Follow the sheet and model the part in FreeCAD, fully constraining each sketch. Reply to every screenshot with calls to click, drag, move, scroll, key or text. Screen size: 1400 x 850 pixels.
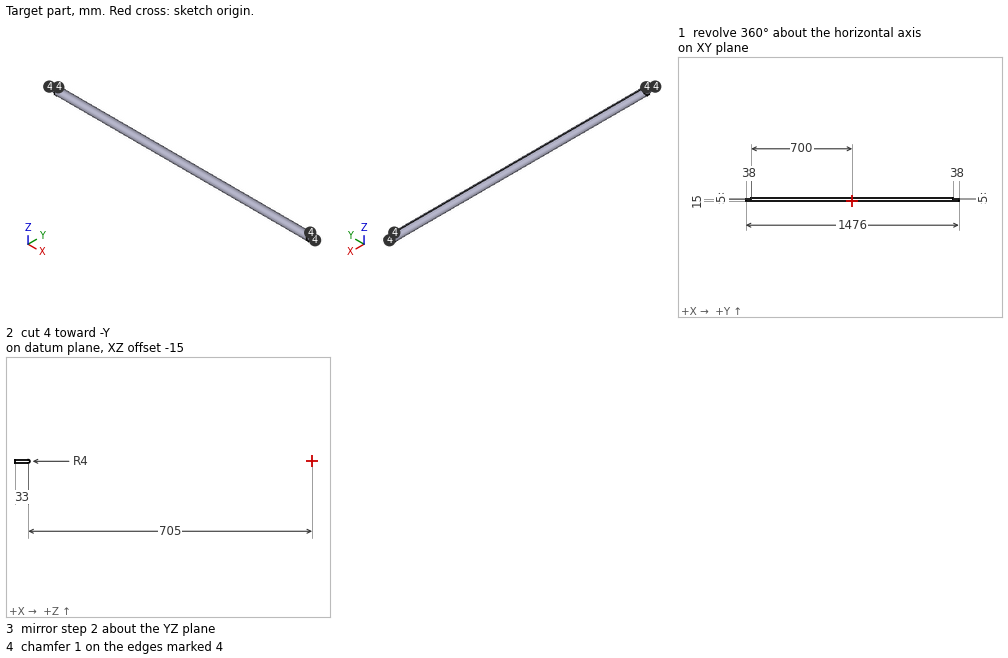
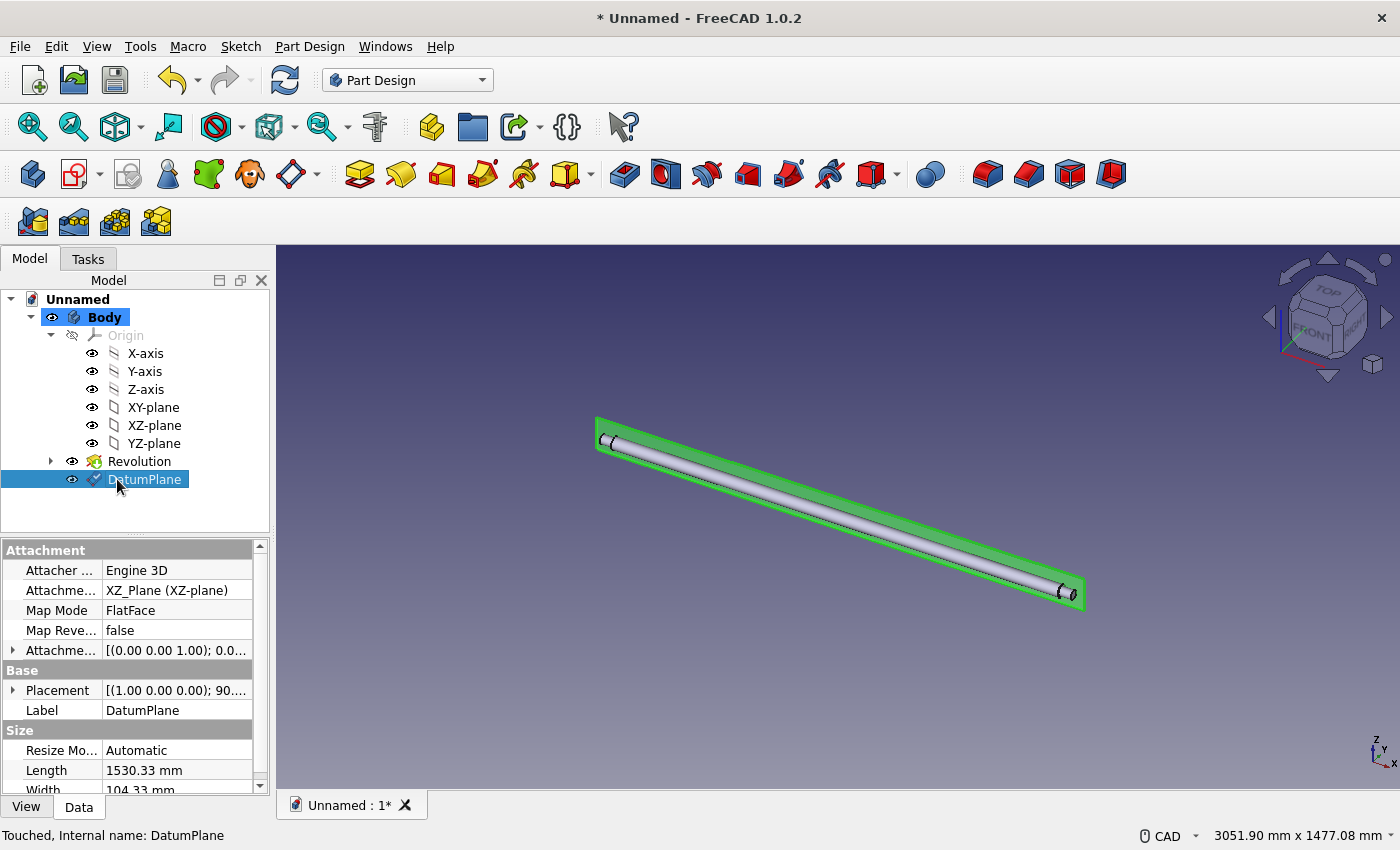
click(74, 174)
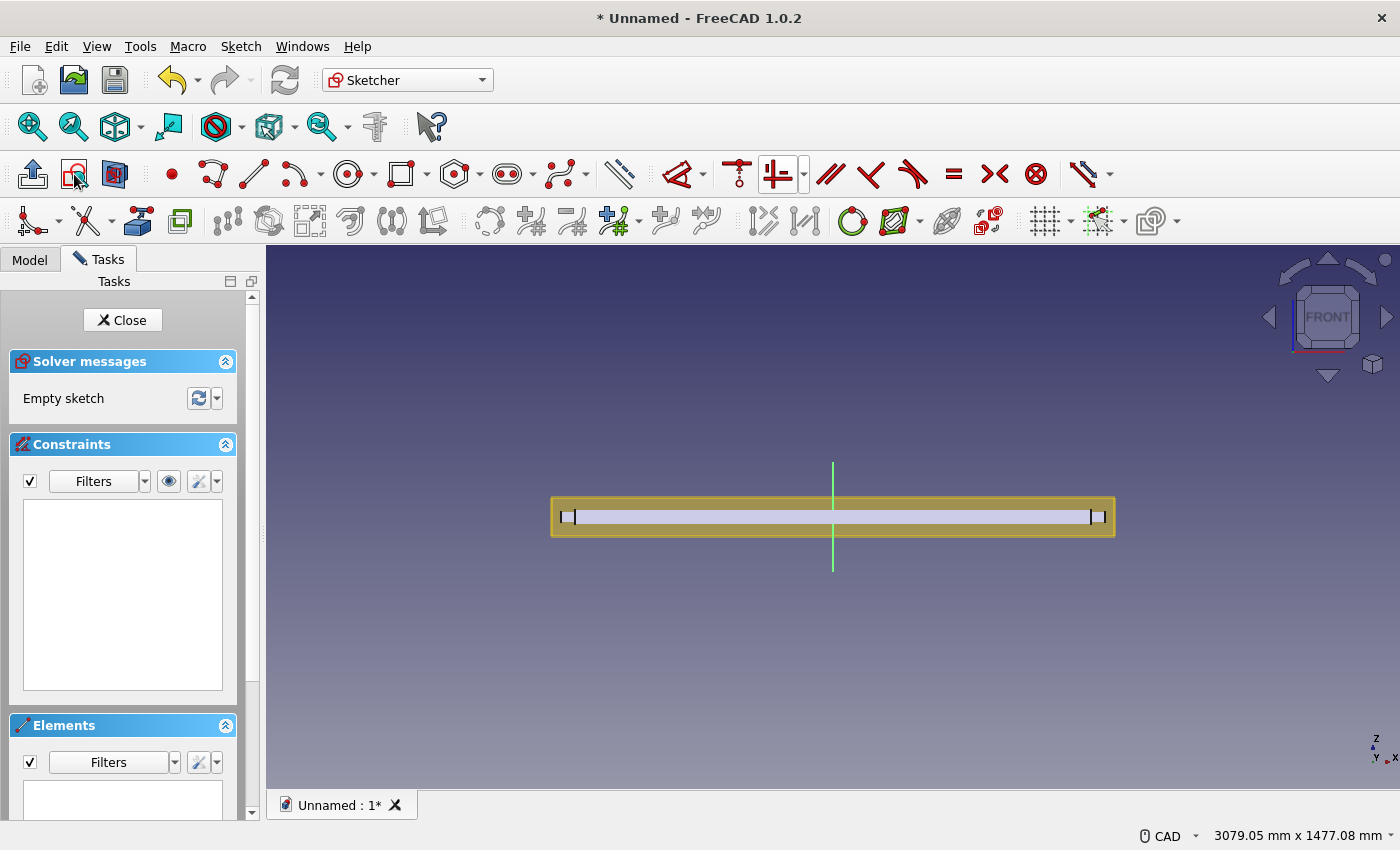
click(115, 174)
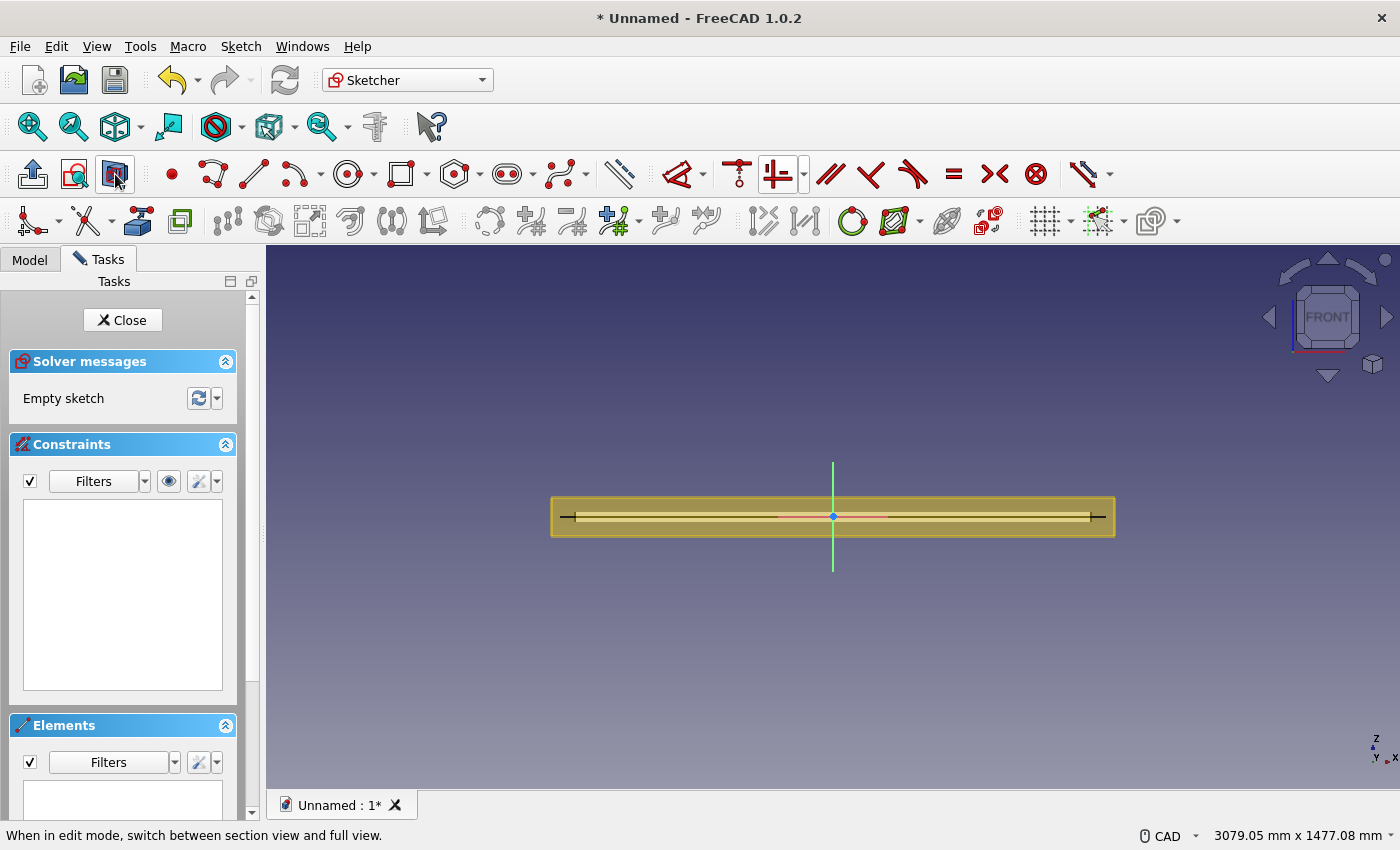
scroll(558, 517, up, 15)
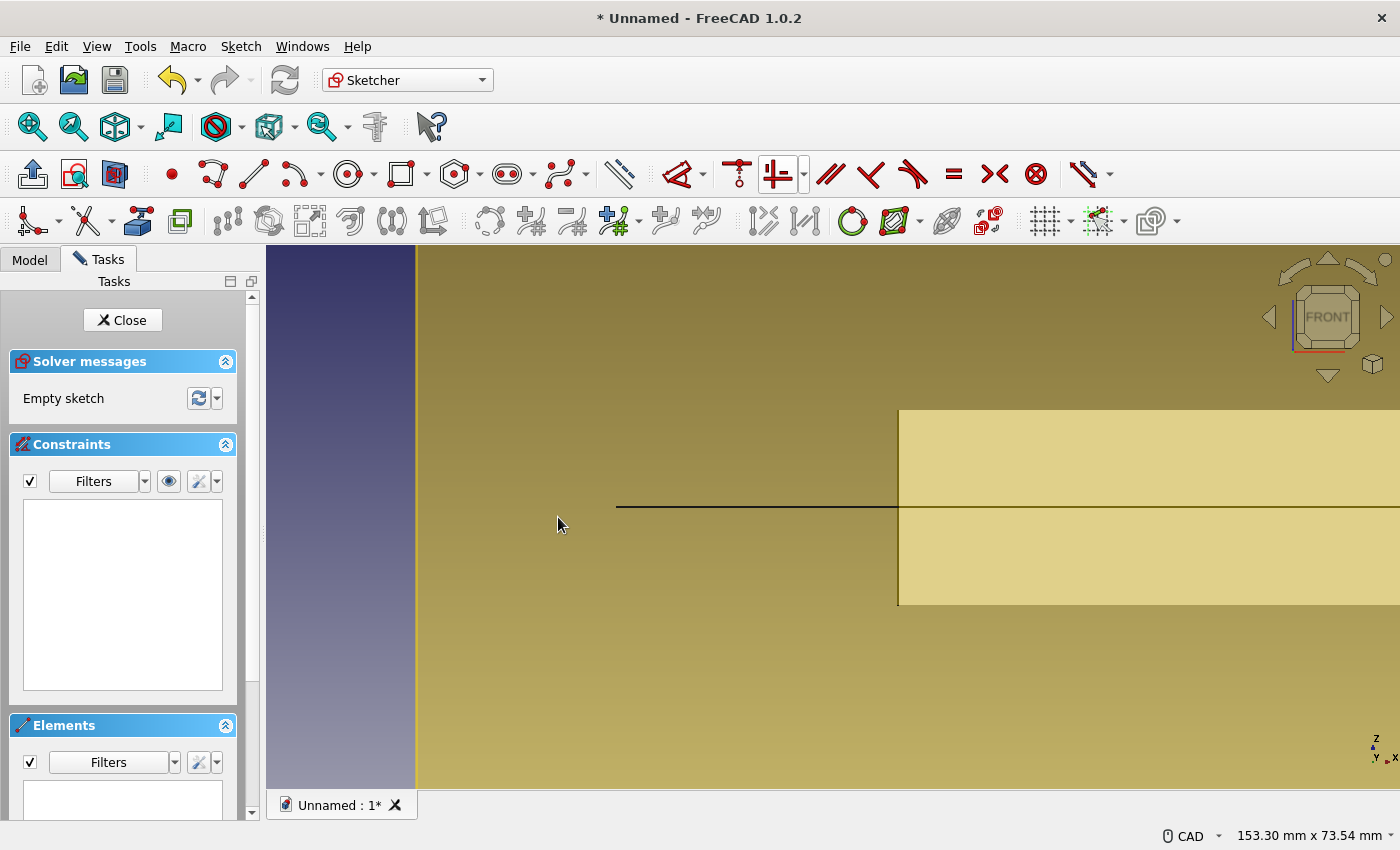
scroll(746, 500, up, 4)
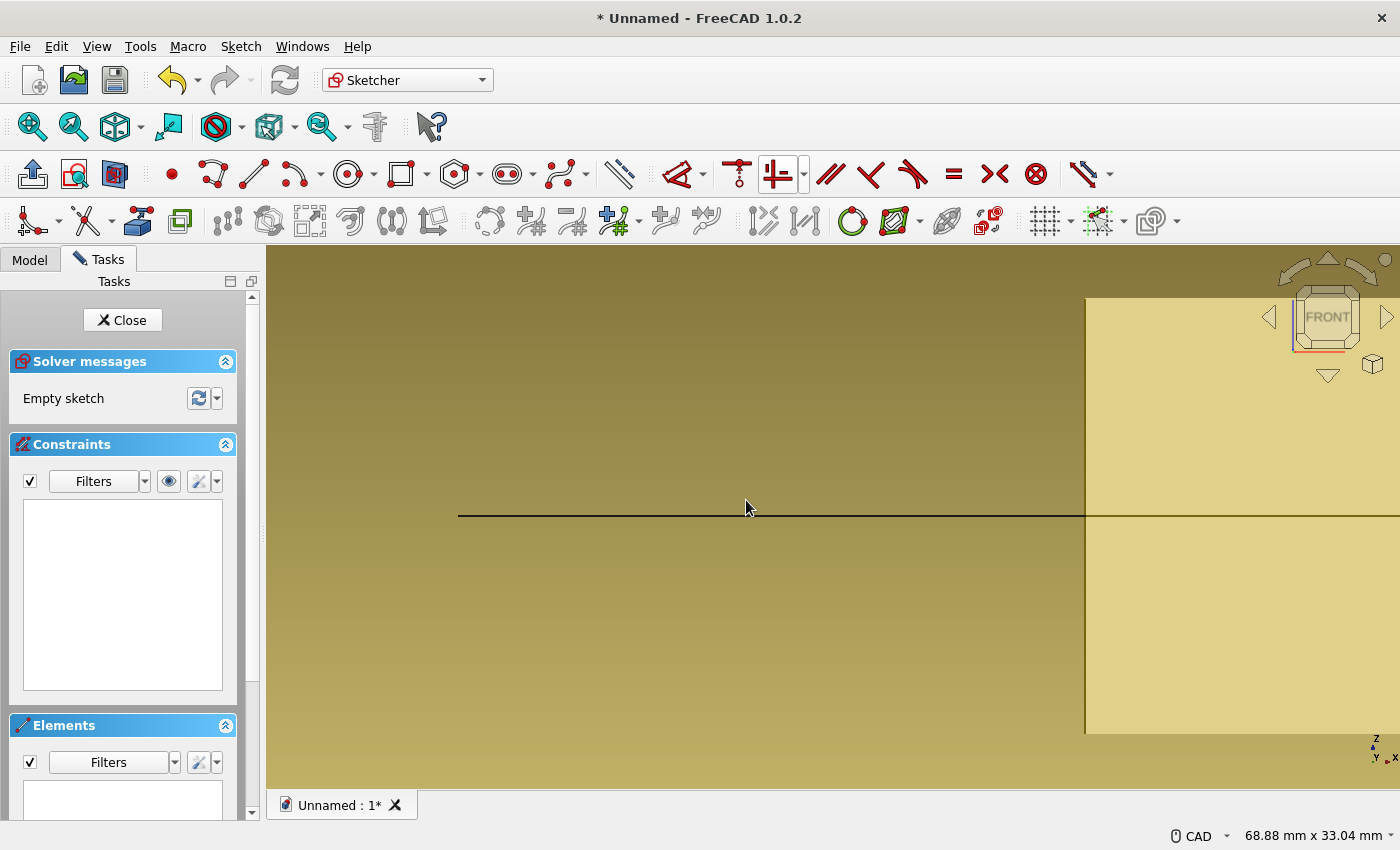
click(213, 174)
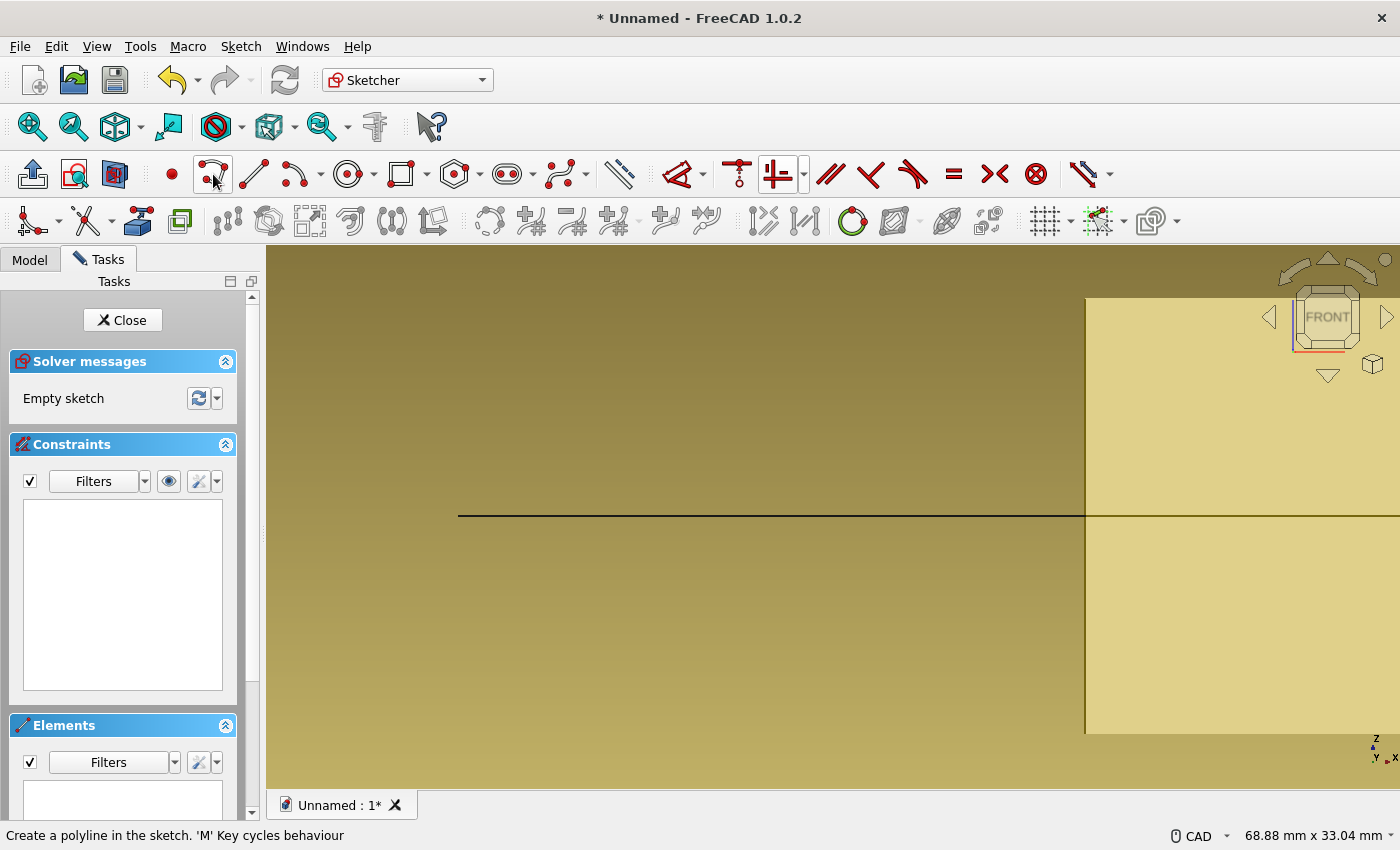
click(1002, 582)
click(459, 582)
click(459, 450)
click(1002, 450)
right_click(1002, 450)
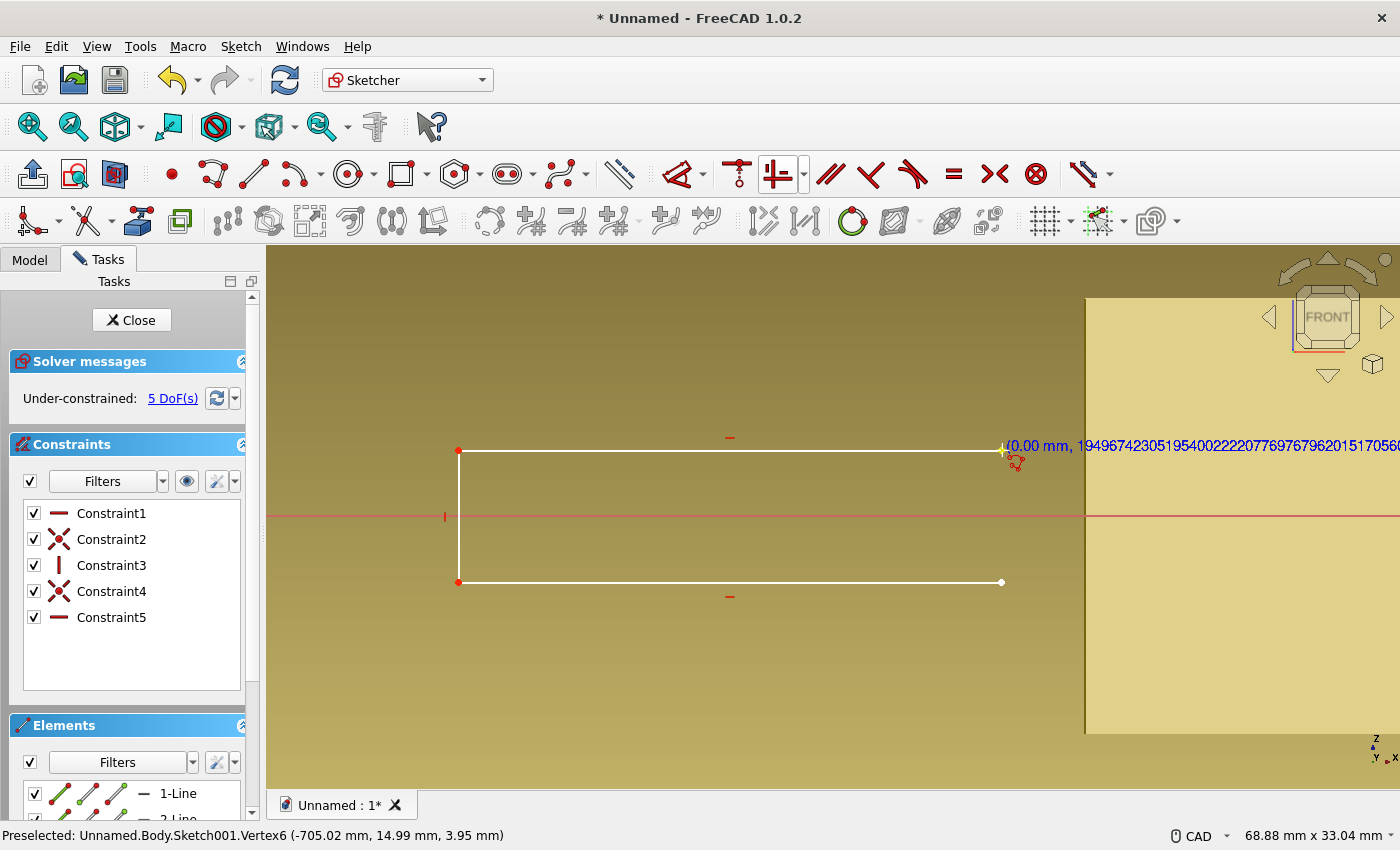
key(g)
key(3)
key(a)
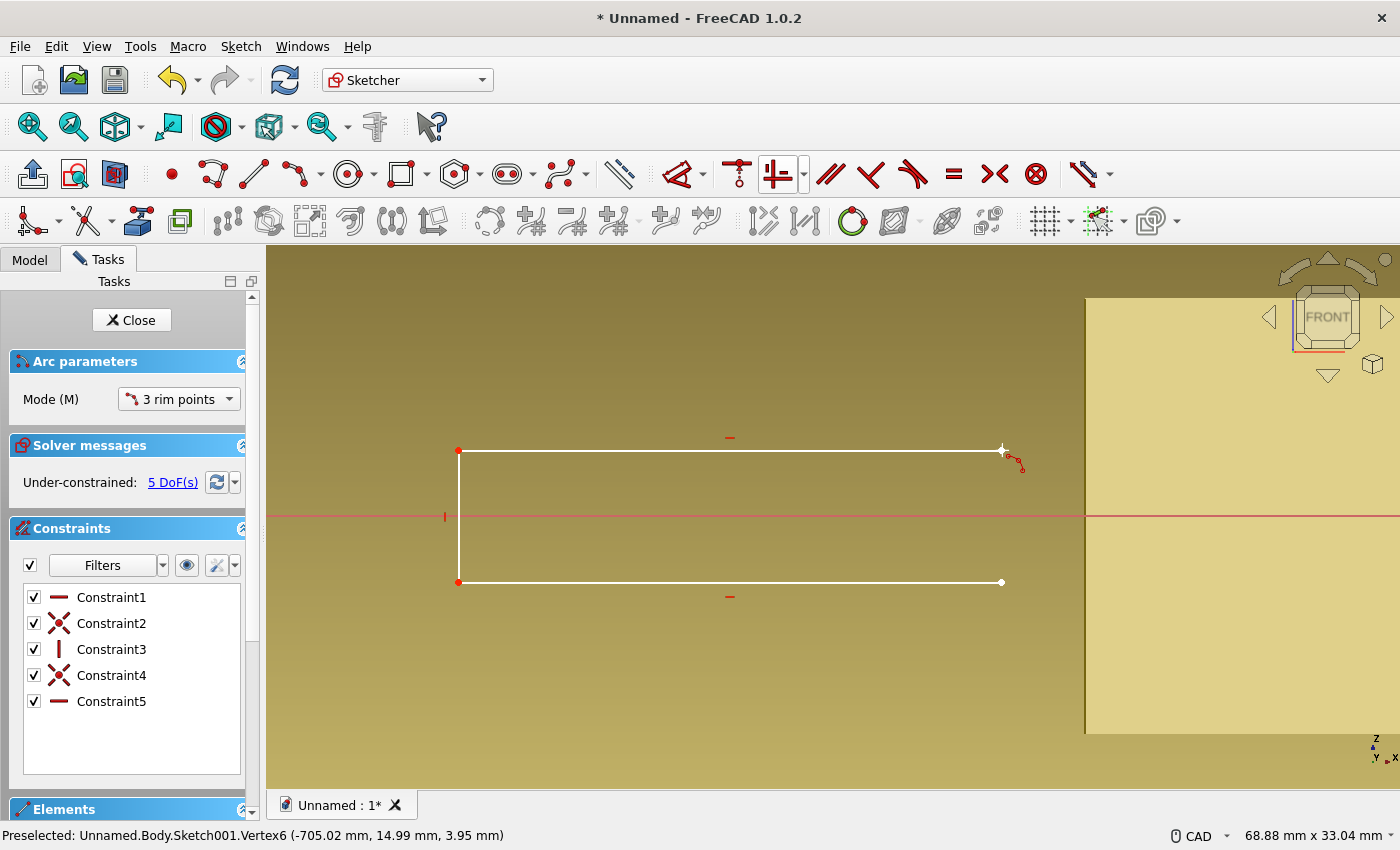
click(1002, 451)
click(1002, 583)
click(1065, 536)
key(Escape)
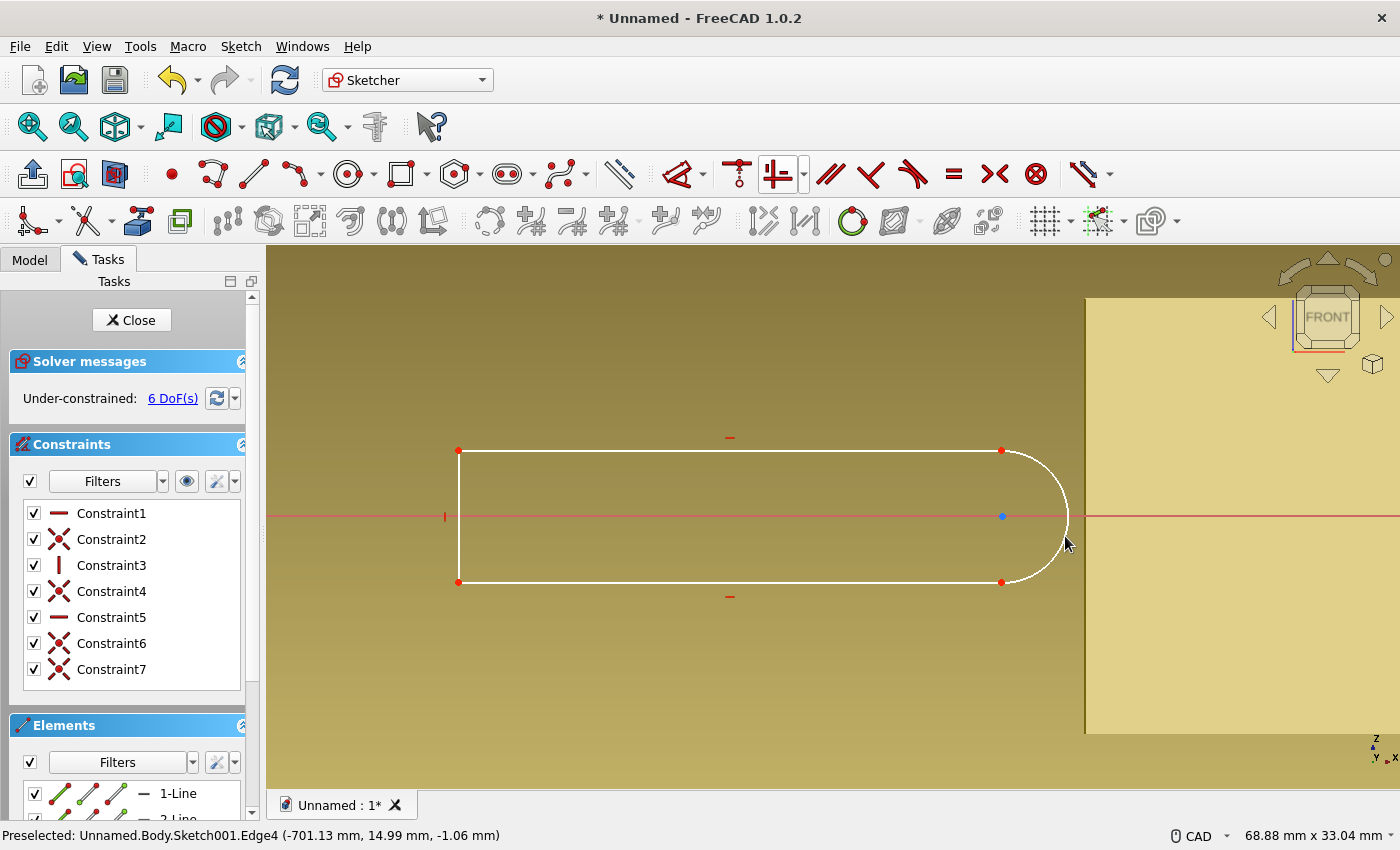
click(839, 583)